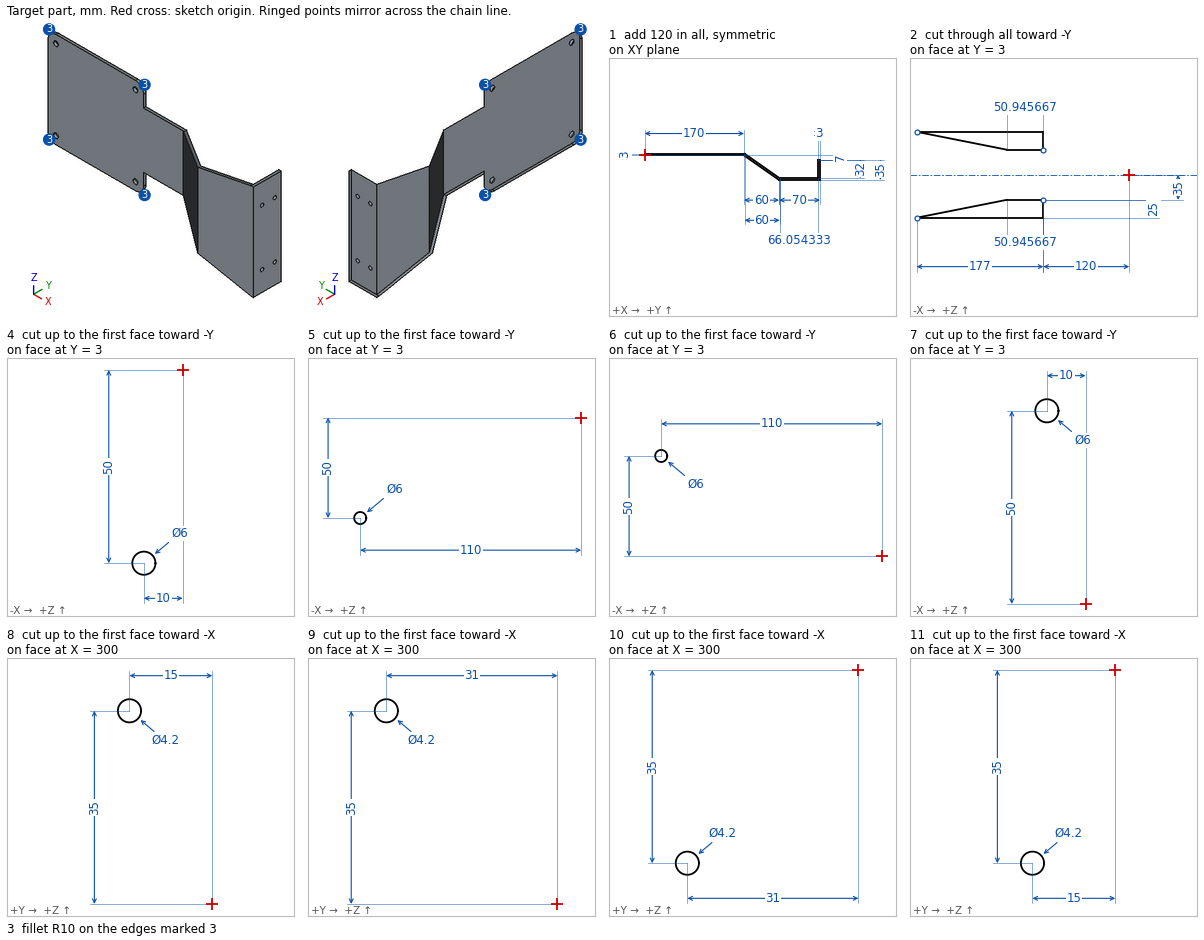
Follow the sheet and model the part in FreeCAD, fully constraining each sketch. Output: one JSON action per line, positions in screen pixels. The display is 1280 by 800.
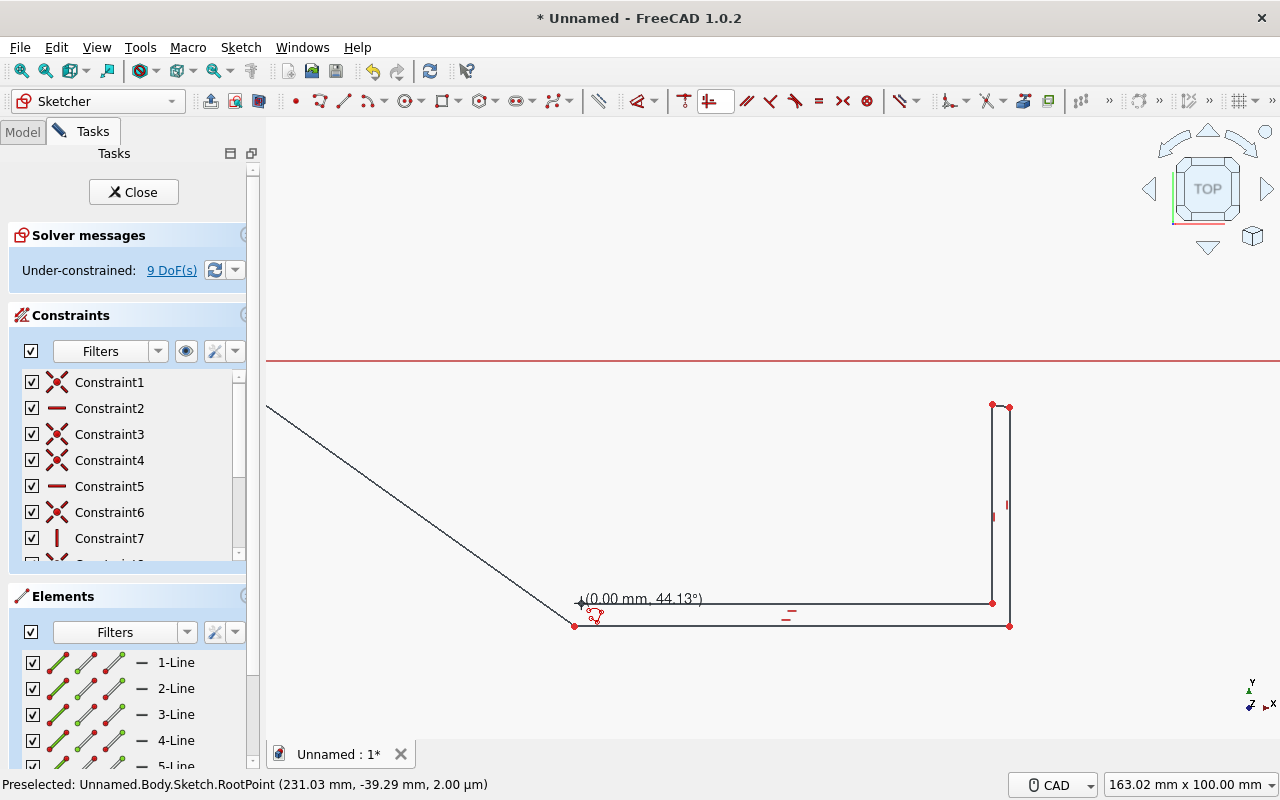
{"action": "scroll", "coordinate": [975, 405], "scroll_direction": "down", "scroll_amount": 6}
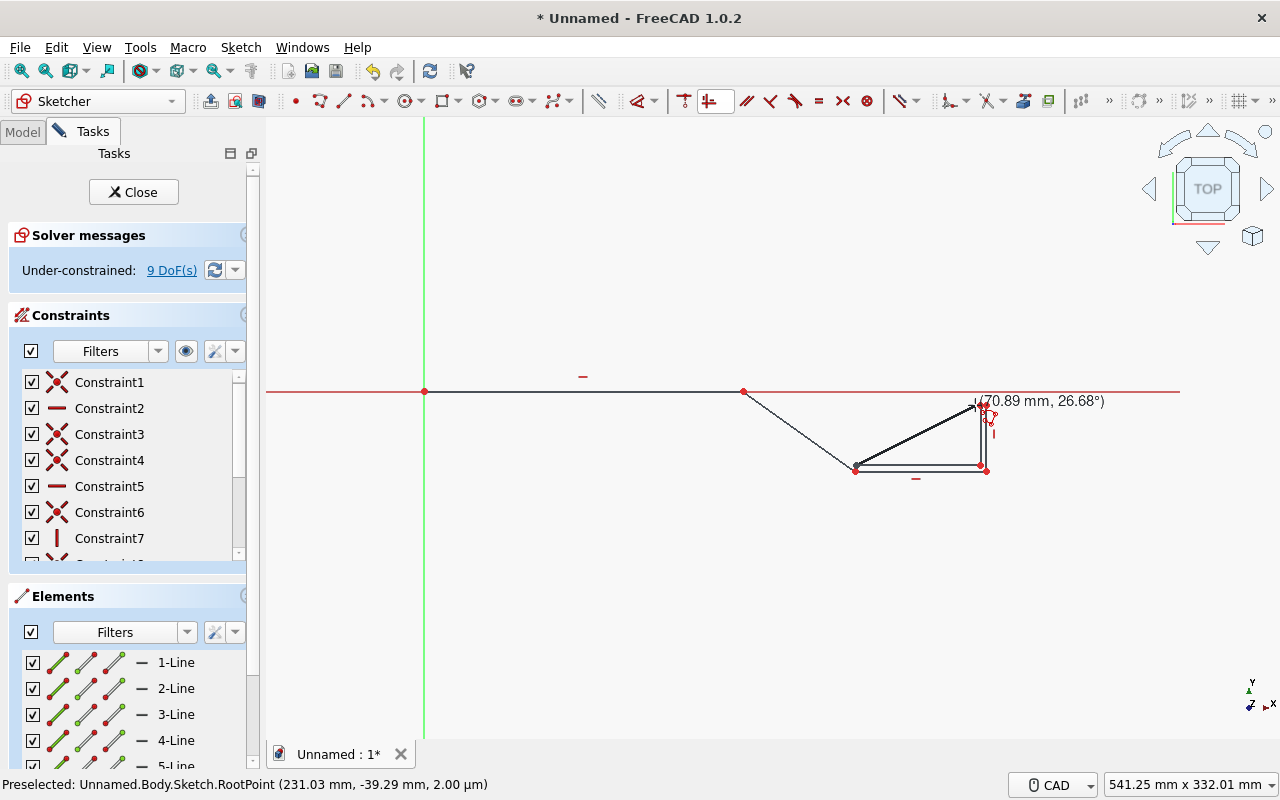
{"action": "scroll", "coordinate": [745, 386], "scroll_direction": "up", "scroll_amount": 6}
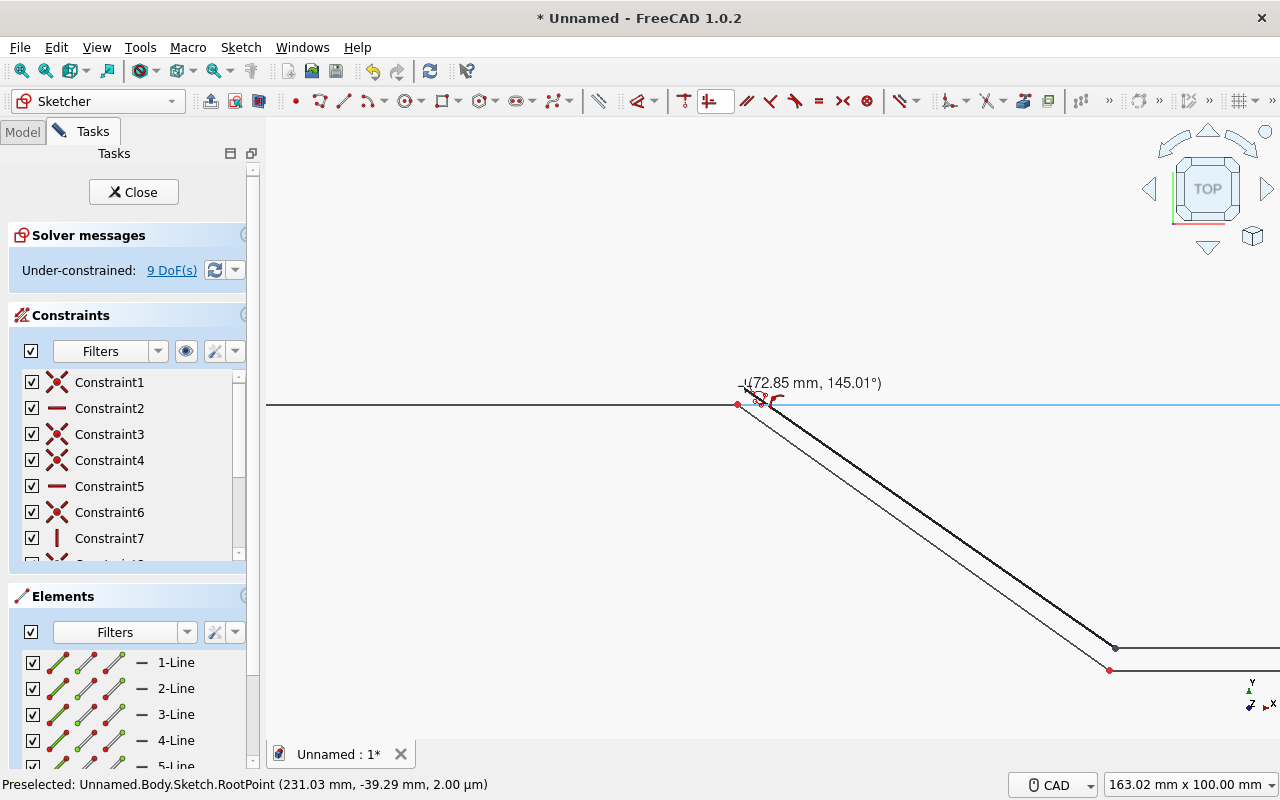
{"action": "left_click", "coordinate": [742, 386]}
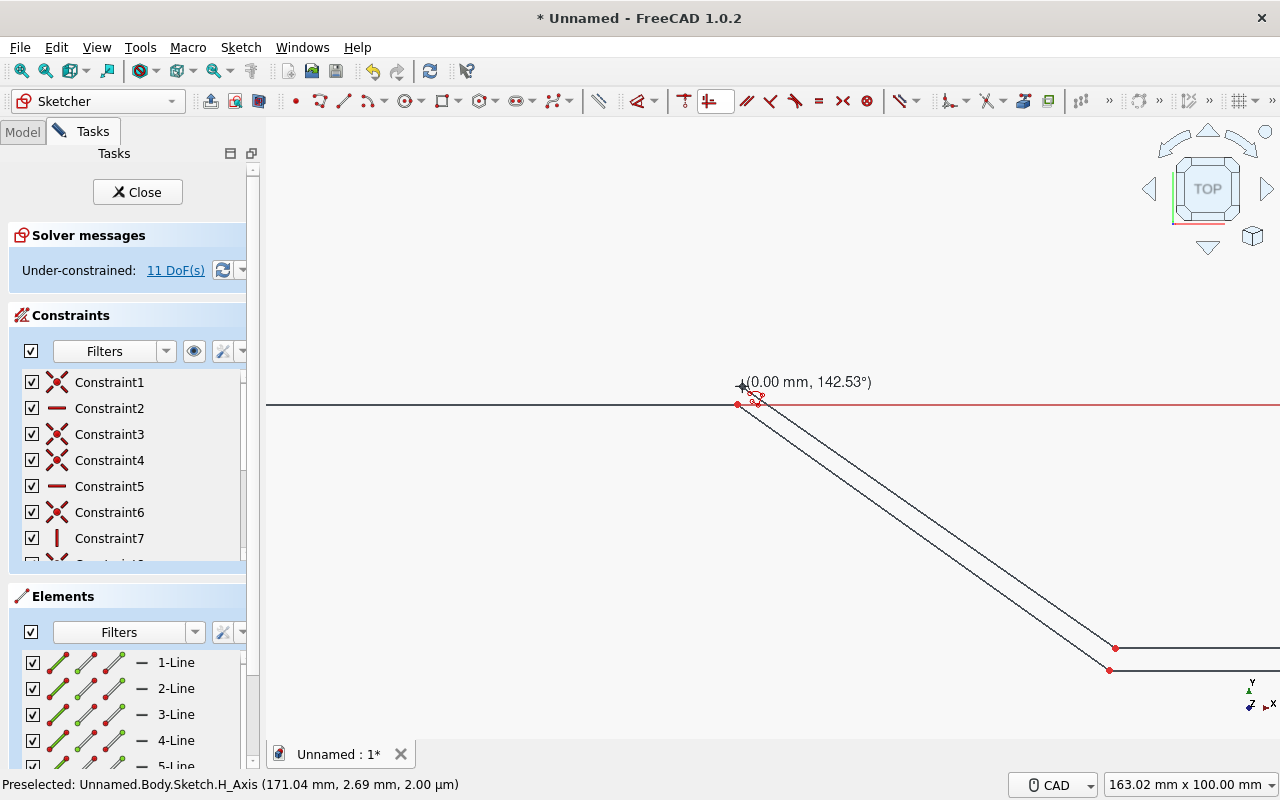
{"action": "scroll", "coordinate": [744, 386], "scroll_direction": "down", "scroll_amount": 6}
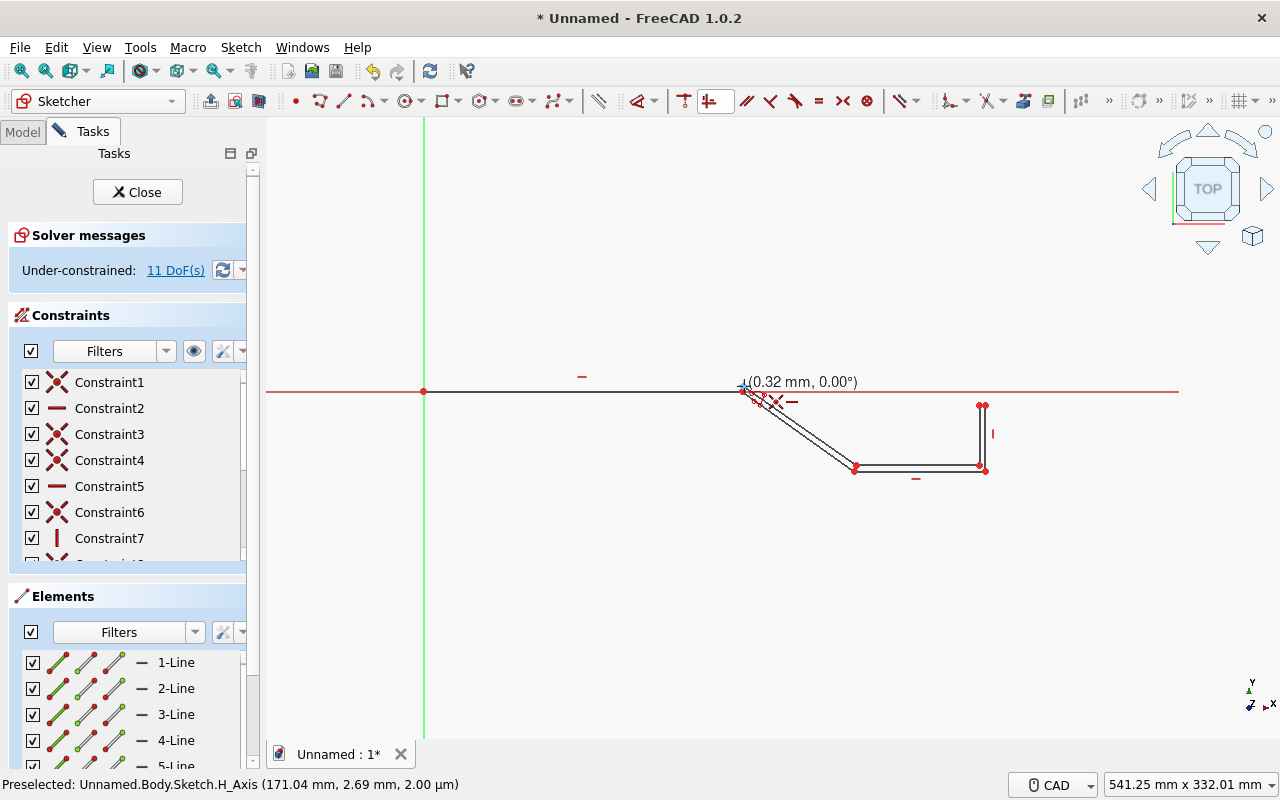
{"action": "scroll", "coordinate": [424, 386], "scroll_direction": "up", "scroll_amount": 6}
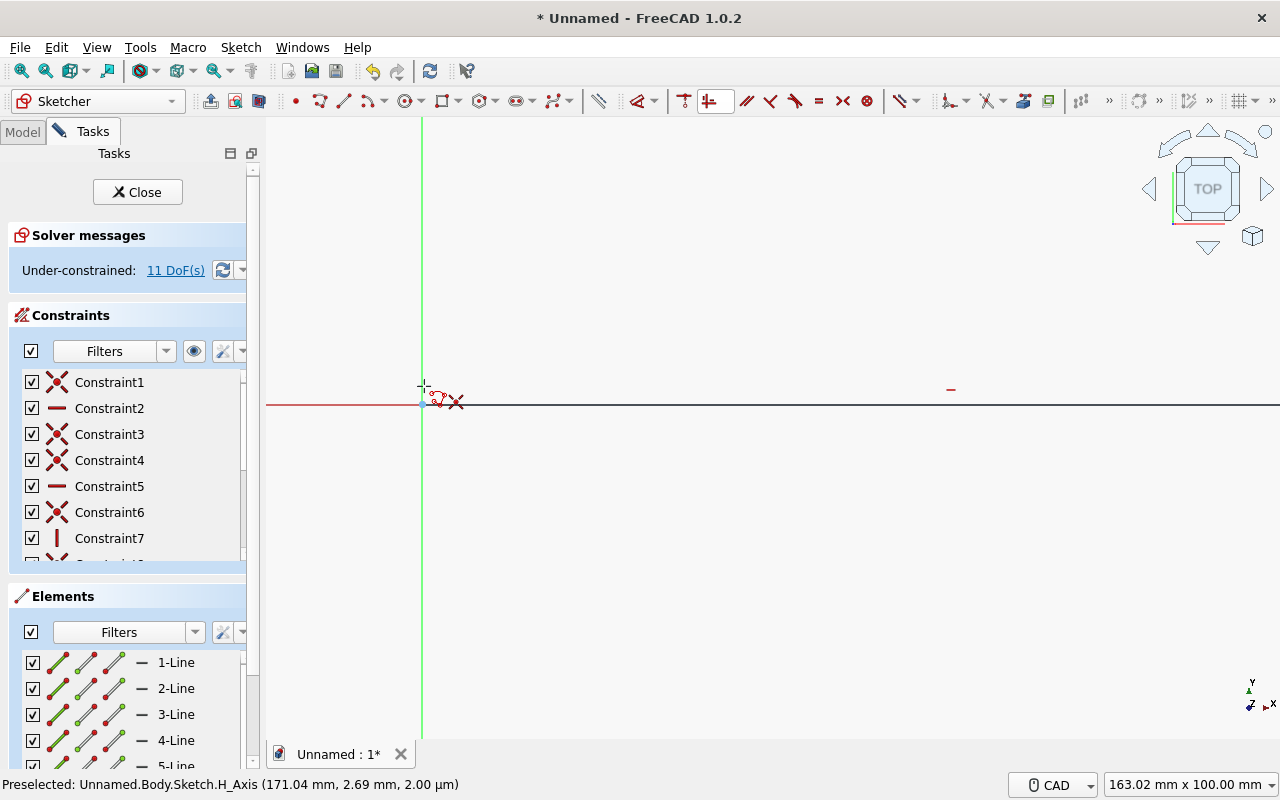
{"action": "left_click", "coordinate": [431, 386]}
{"action": "left_click", "coordinate": [422, 405]}
{"action": "key", "text": "Escape"}
{"action": "key", "text": "Escape"}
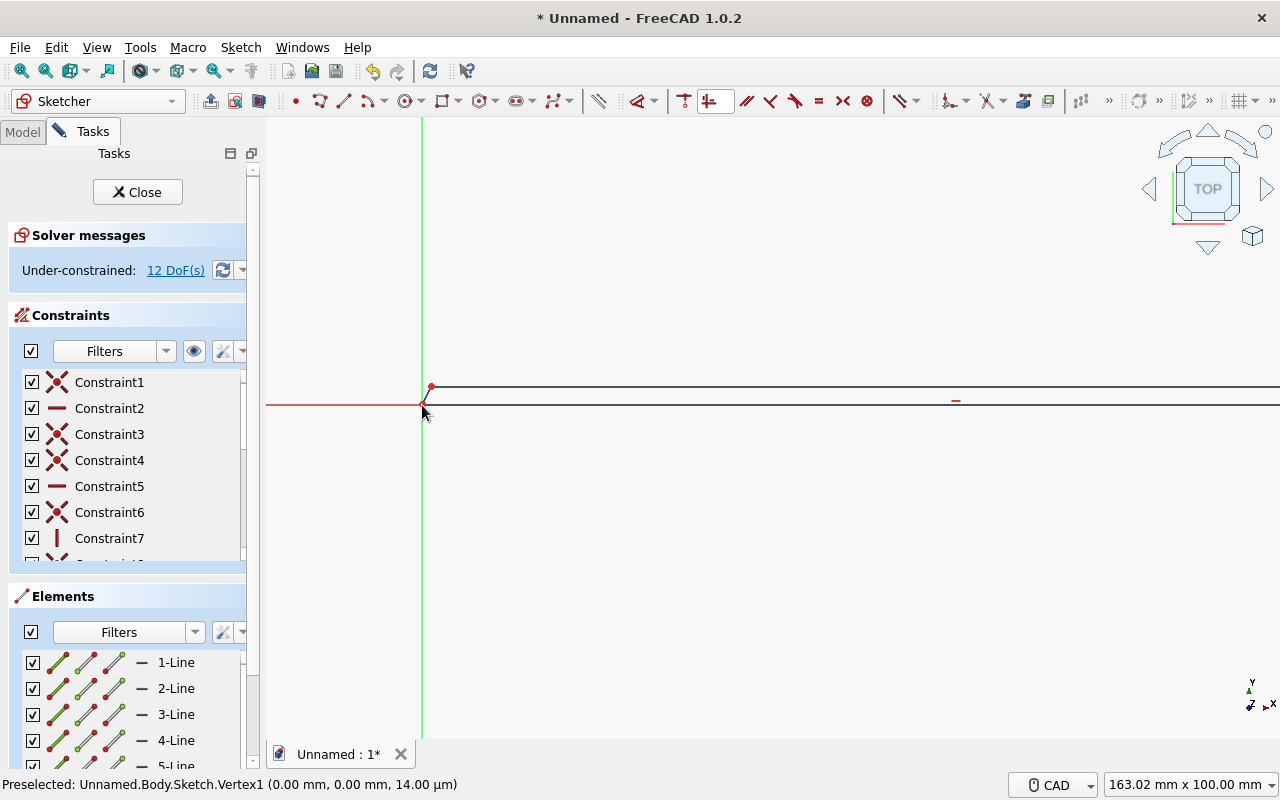
{"action": "scroll", "coordinate": [424, 386], "scroll_direction": "down", "scroll_amount": 6}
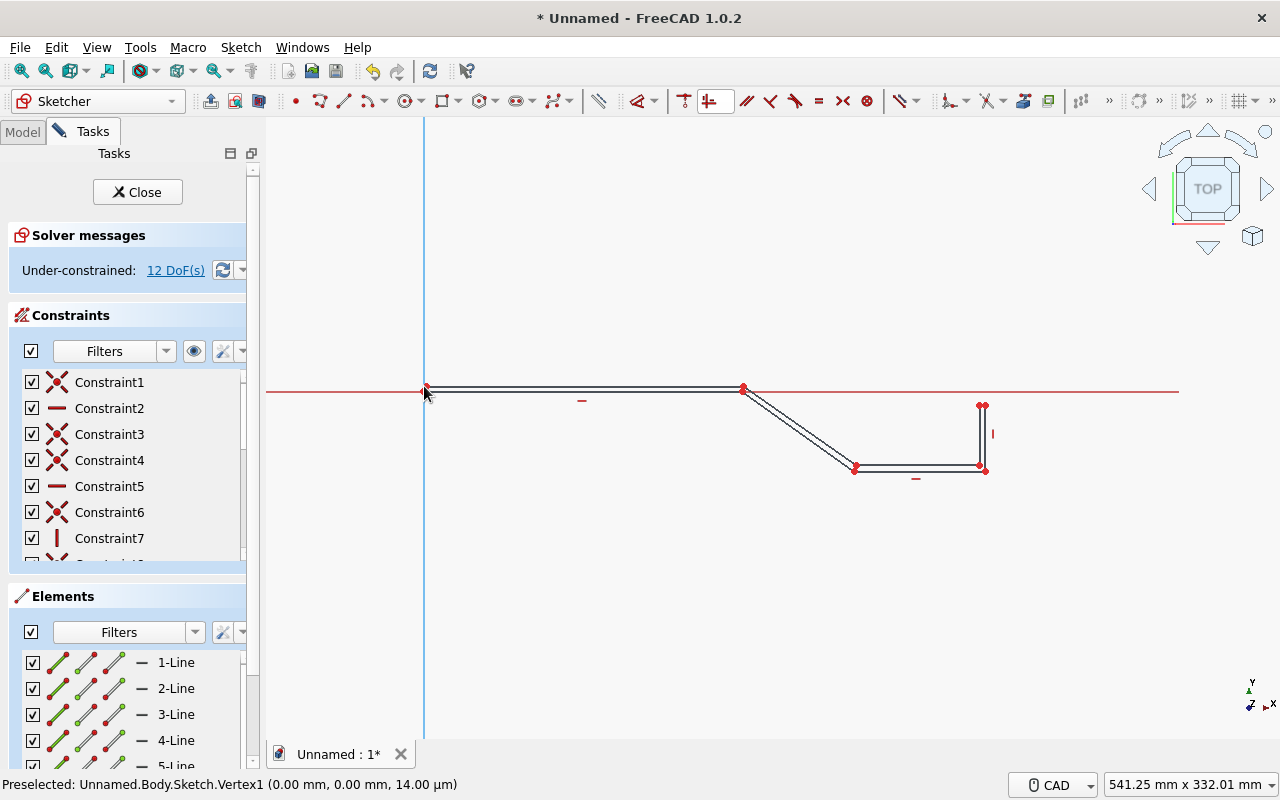
{"action": "scroll", "coordinate": [983, 406], "scroll_direction": "up", "scroll_amount": 9}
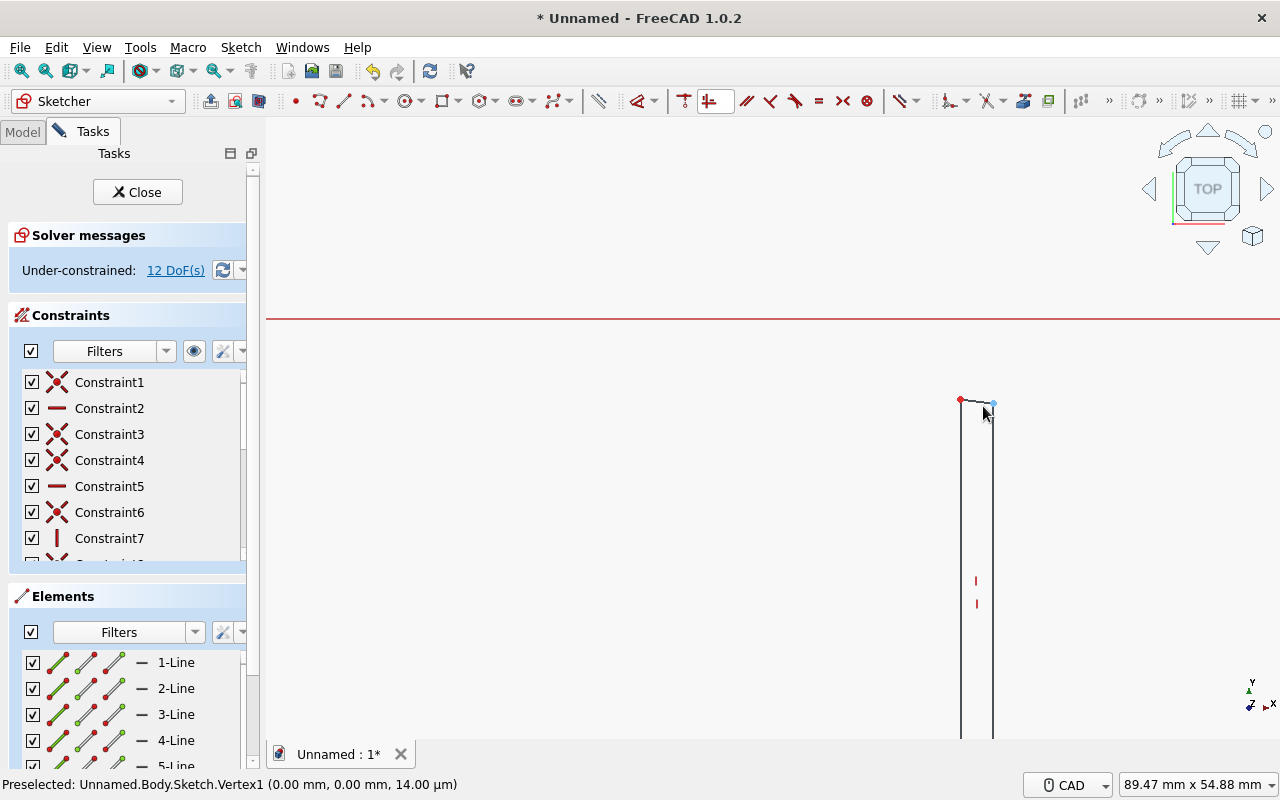
{"action": "left_click", "coordinate": [977, 402]}